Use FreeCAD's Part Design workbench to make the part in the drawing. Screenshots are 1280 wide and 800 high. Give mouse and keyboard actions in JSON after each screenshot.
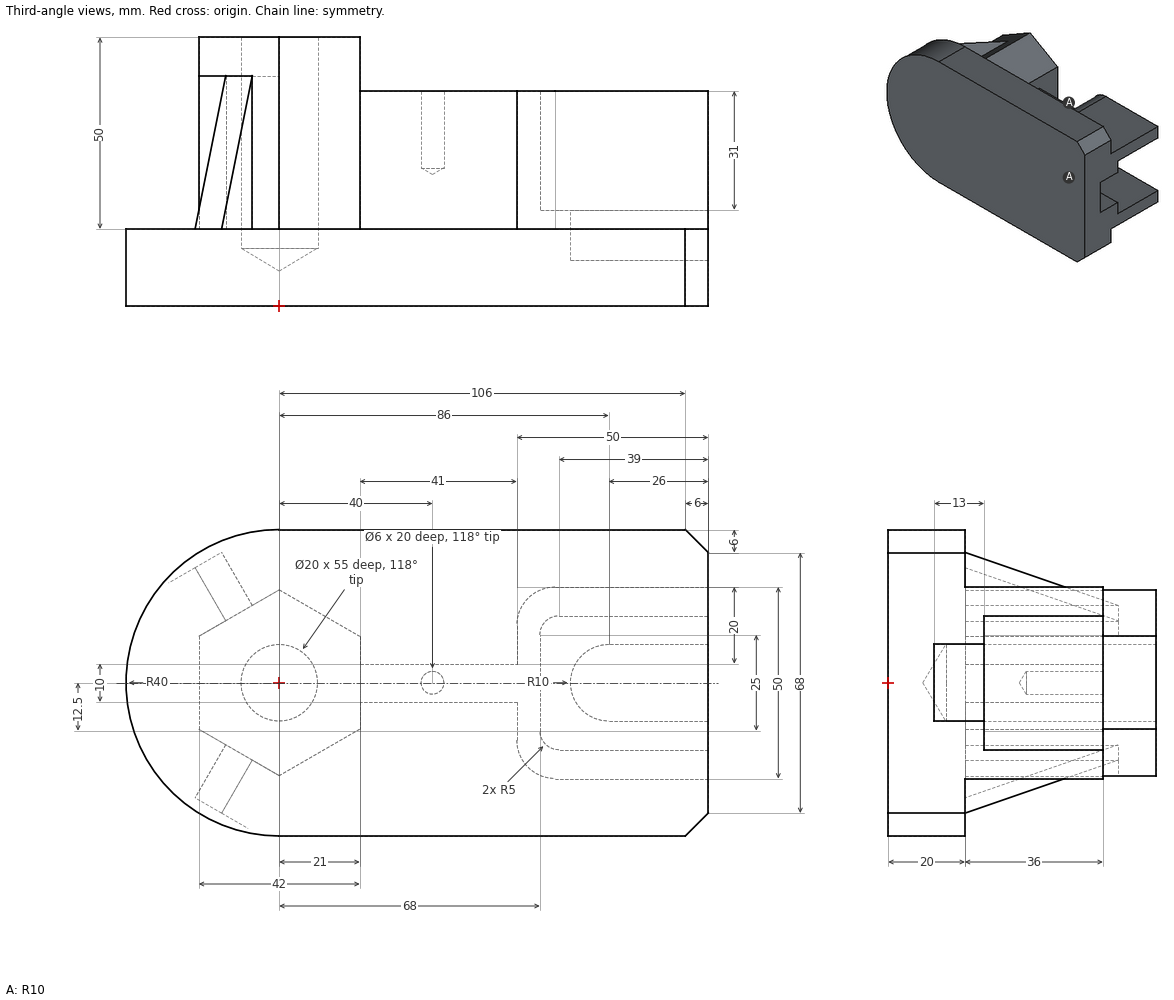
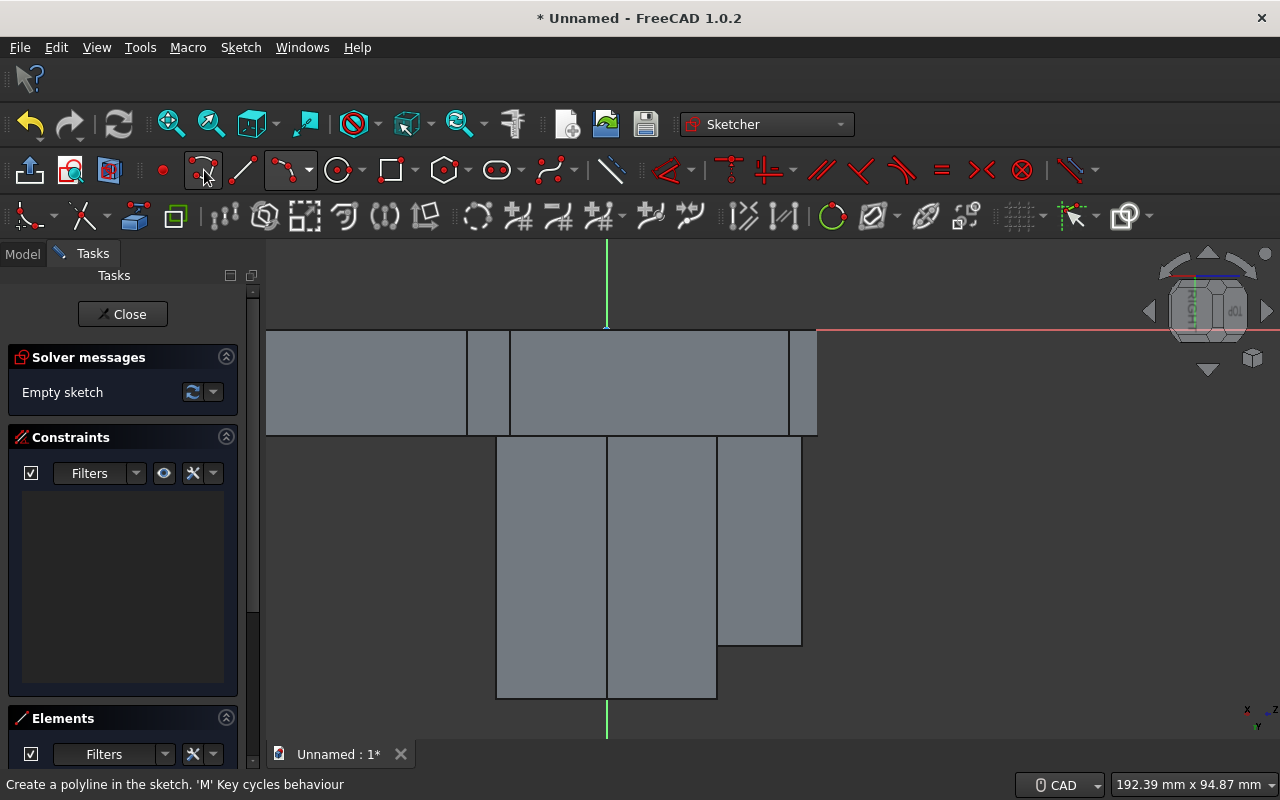
{"action": "left_click", "coordinate": [802, 436]}
{"action": "left_click", "coordinate": [717, 646]}
{"action": "left_click", "coordinate": [802, 646]}
{"action": "left_click", "coordinate": [802, 437]}
{"action": "key", "text": "Escape"}
{"action": "key", "text": "Escape"}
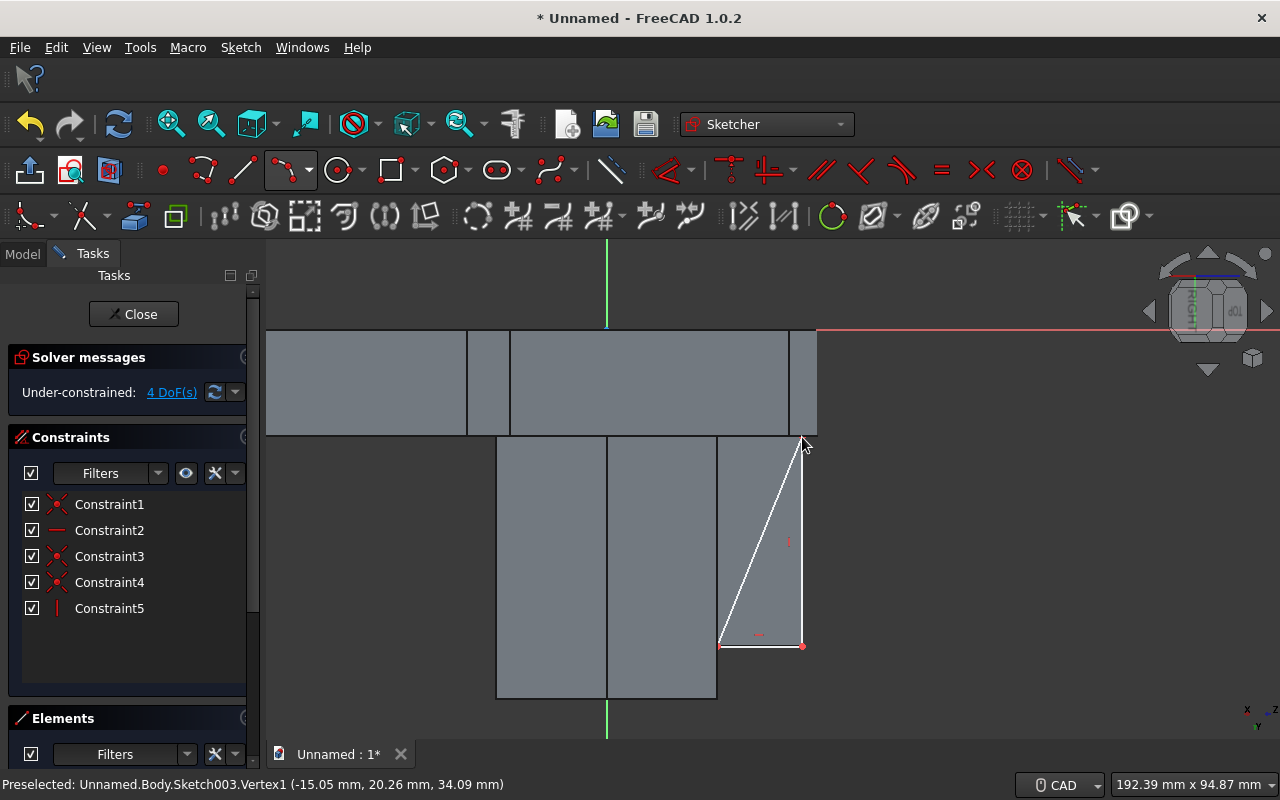
{"action": "left_click", "coordinate": [666, 170]}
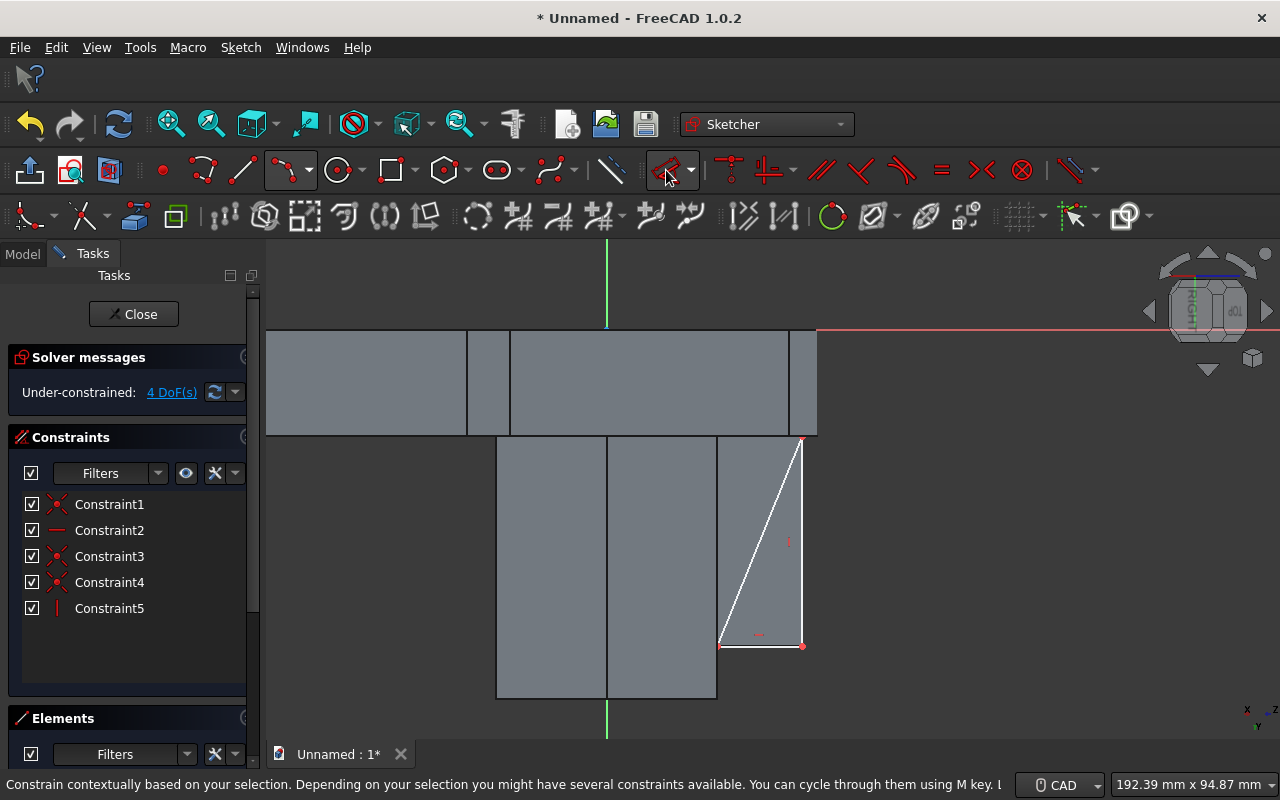
{"action": "left_click", "coordinate": [742, 647]}
{"action": "left_click", "coordinate": [760, 681]}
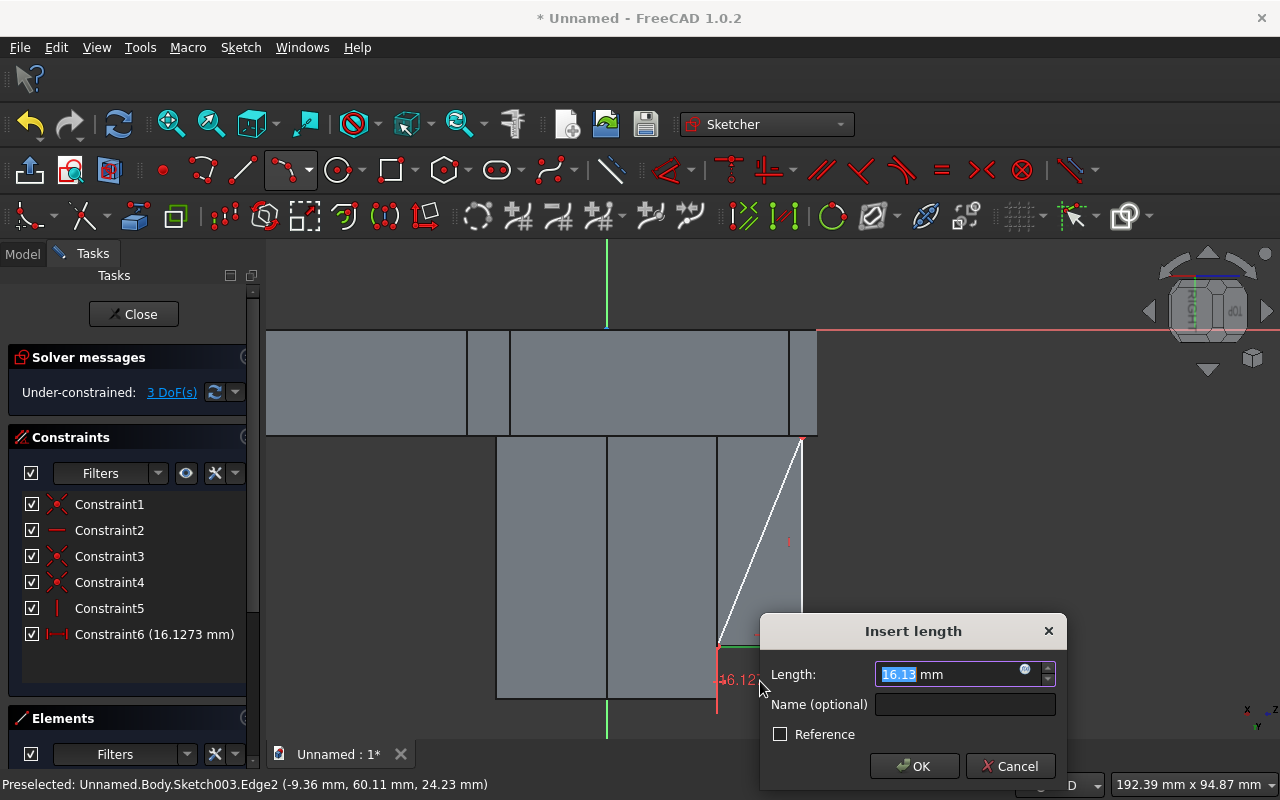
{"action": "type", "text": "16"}
{"action": "key", "text": "Return"}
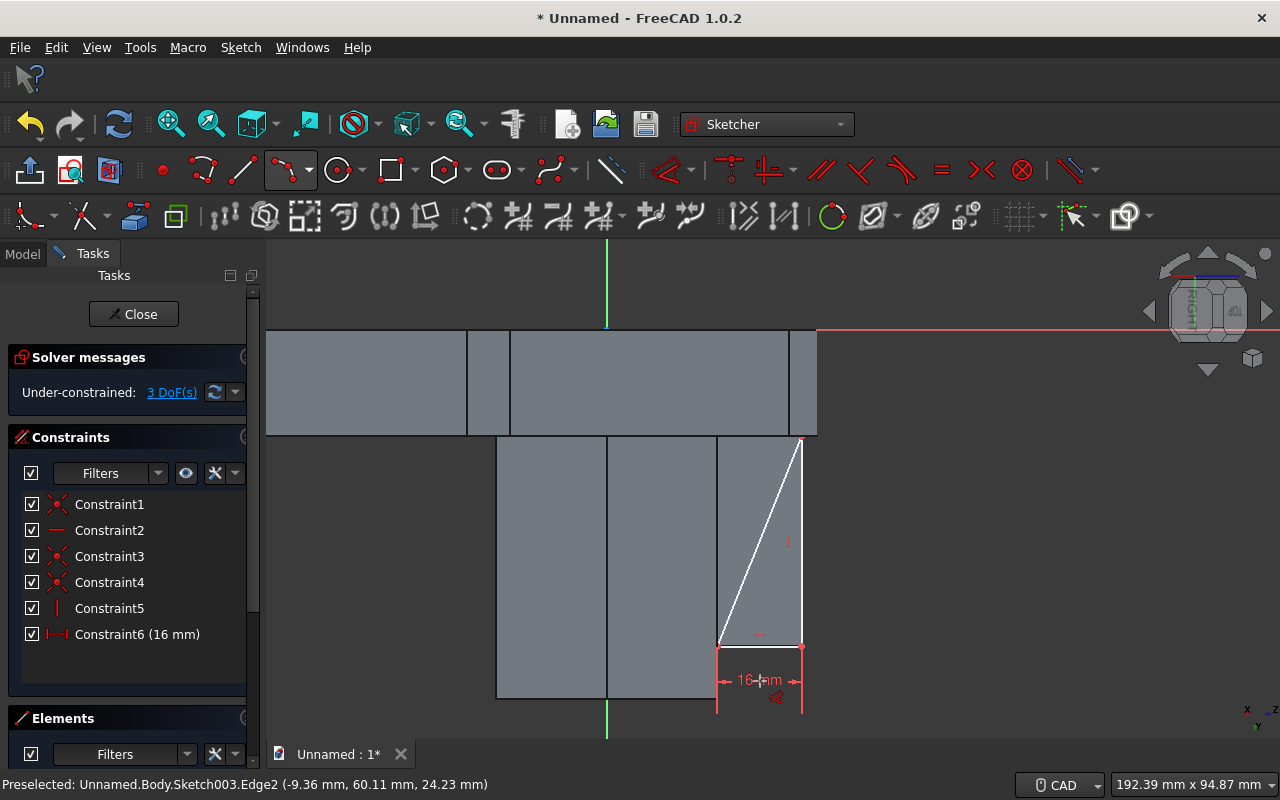
{"action": "left_click", "coordinate": [802, 584]}
{"action": "left_click", "coordinate": [836, 542]}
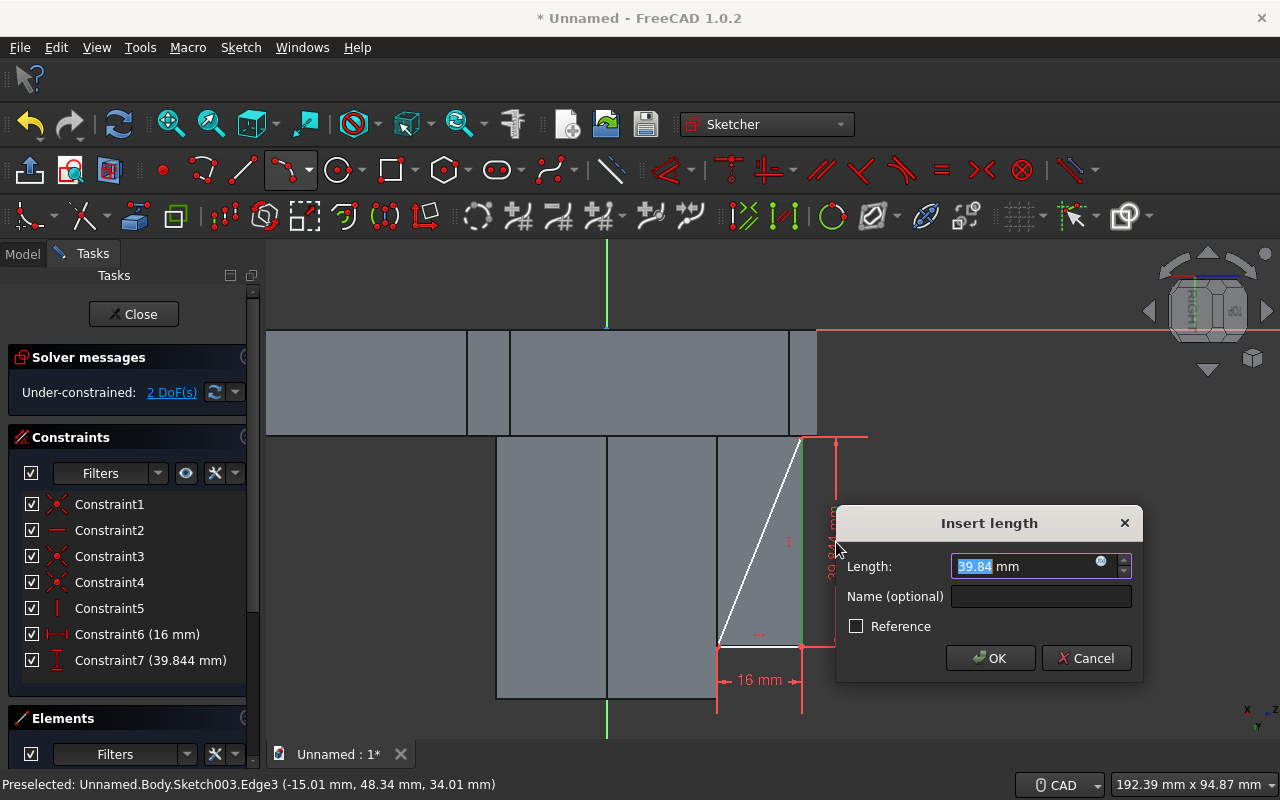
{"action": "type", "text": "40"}
{"action": "key", "text": "Return"}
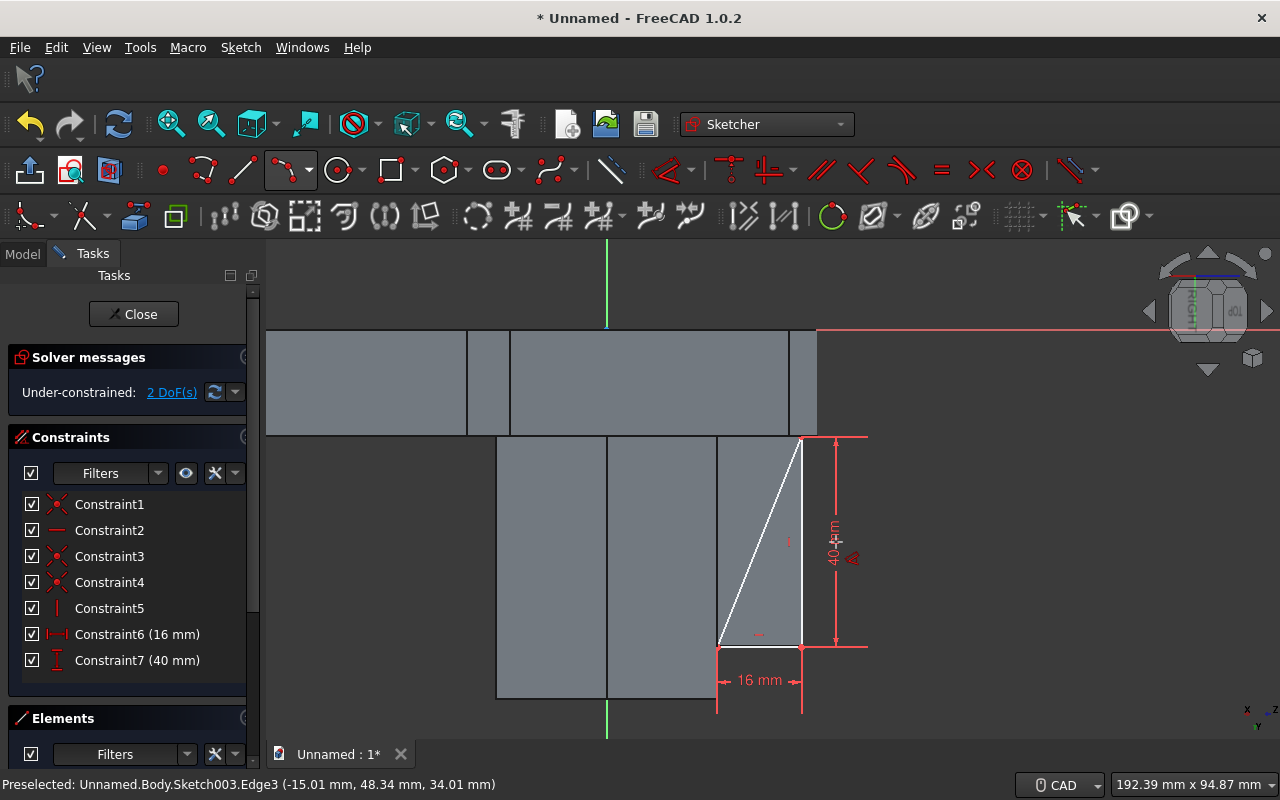
{"action": "left_click", "coordinate": [802, 437]}
{"action": "left_click", "coordinate": [704, 296]}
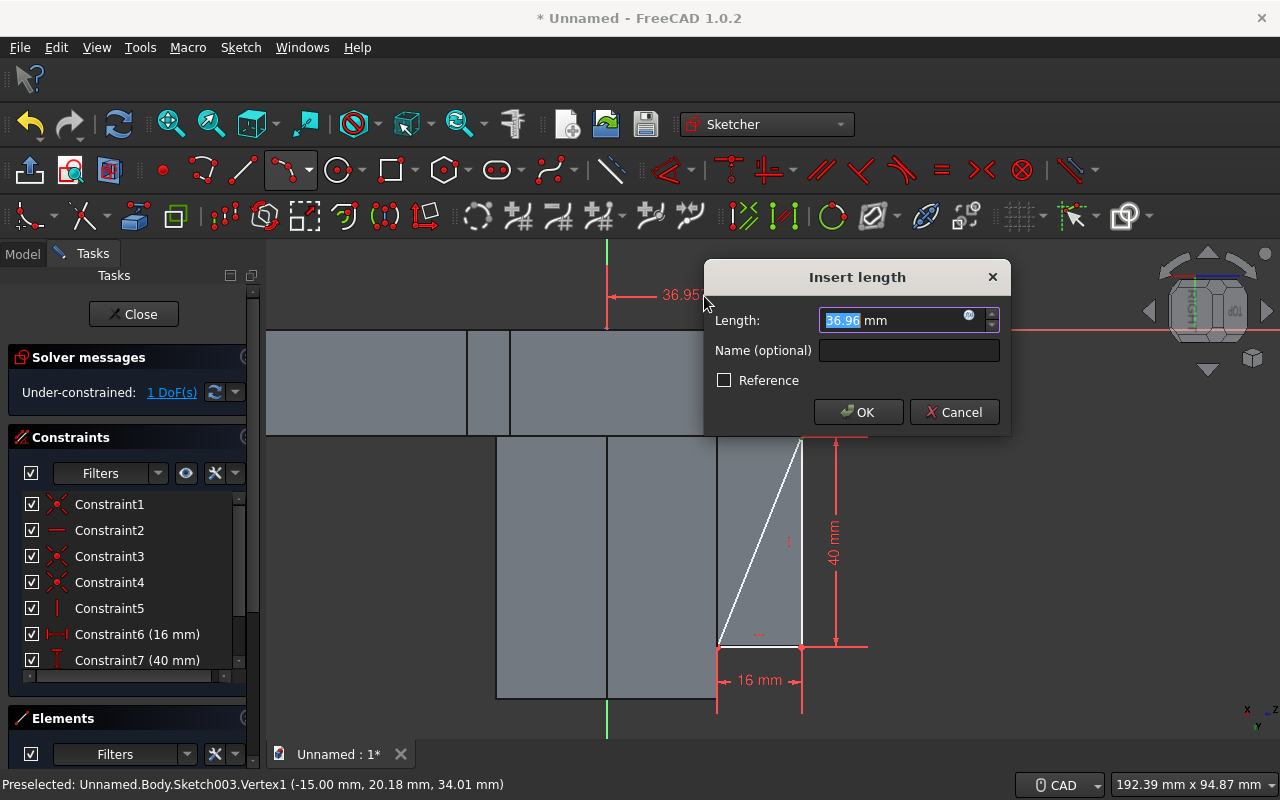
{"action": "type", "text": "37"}
{"action": "key", "text": "Return"}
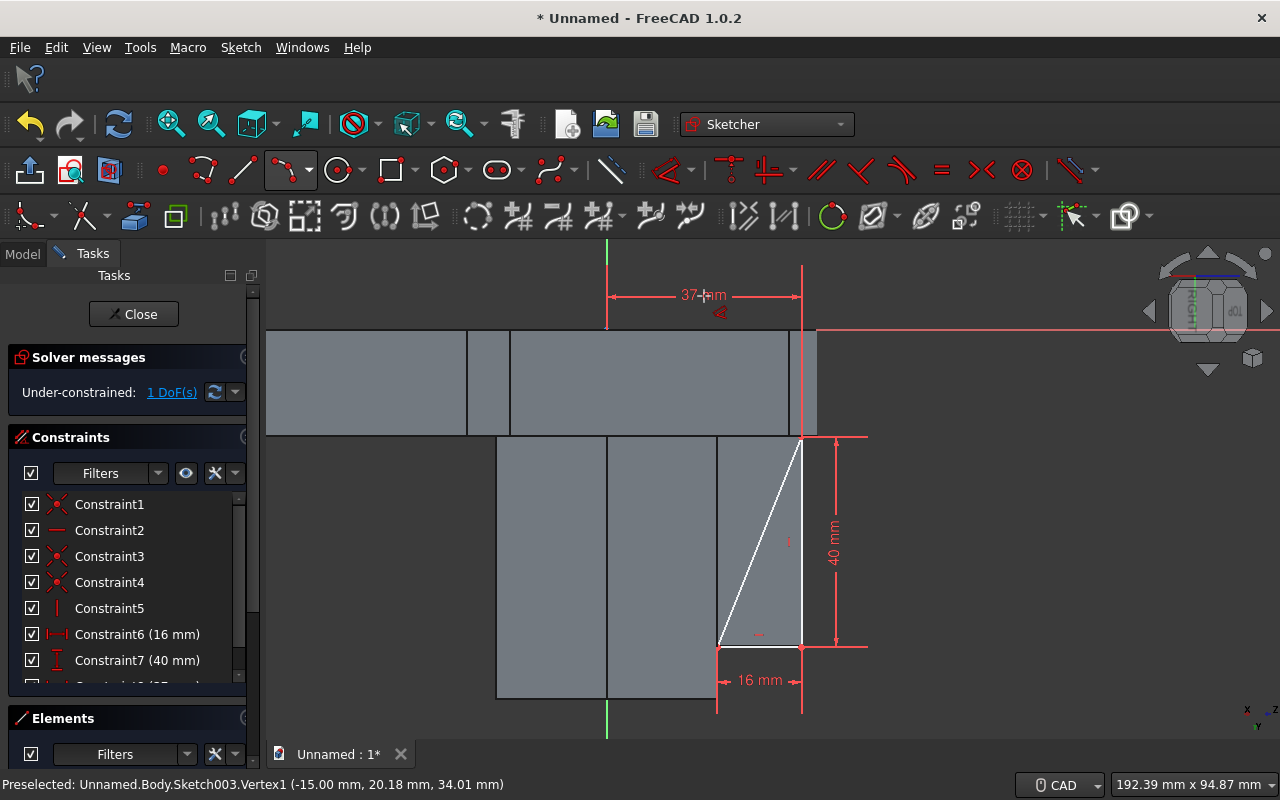
{"action": "left_click", "coordinate": [802, 437]}
{"action": "left_click", "coordinate": [573, 383]}